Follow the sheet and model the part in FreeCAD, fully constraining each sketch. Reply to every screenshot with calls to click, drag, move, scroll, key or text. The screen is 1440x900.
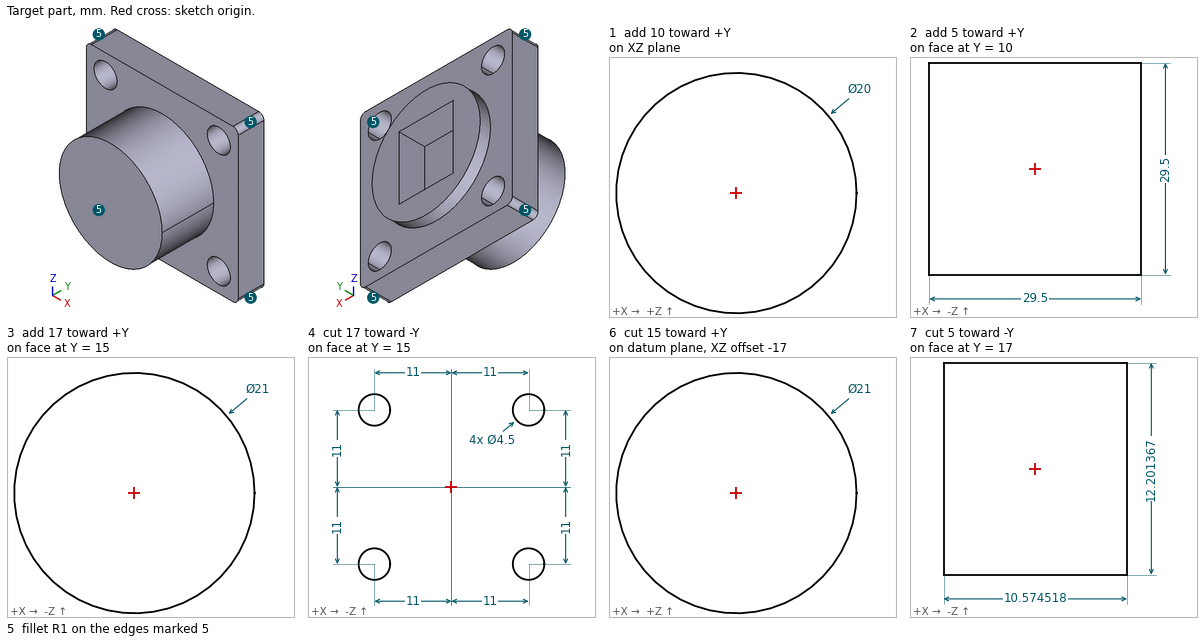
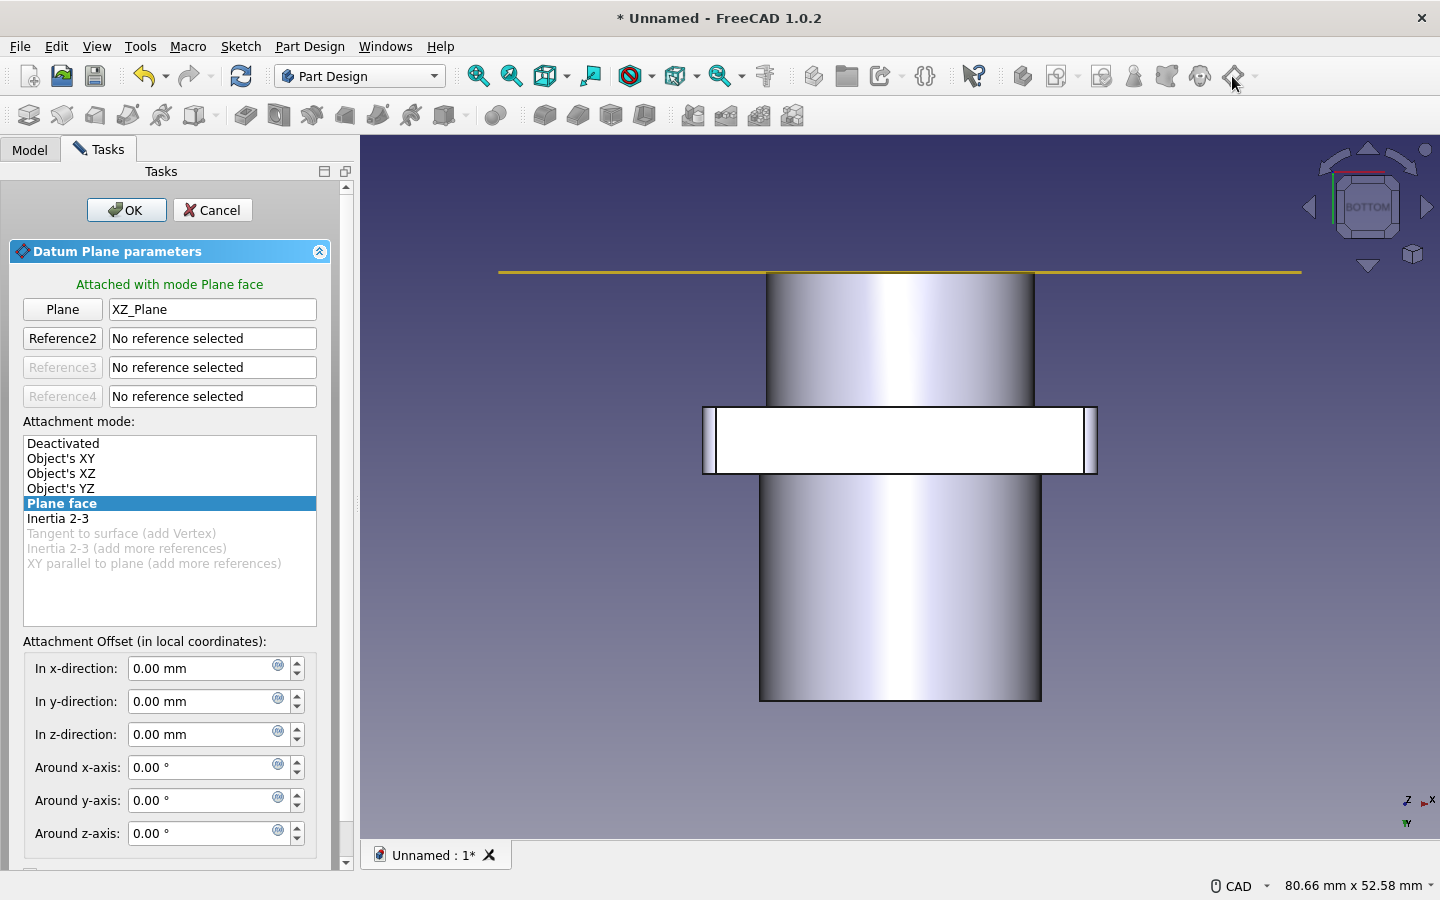
triple_click(210, 734)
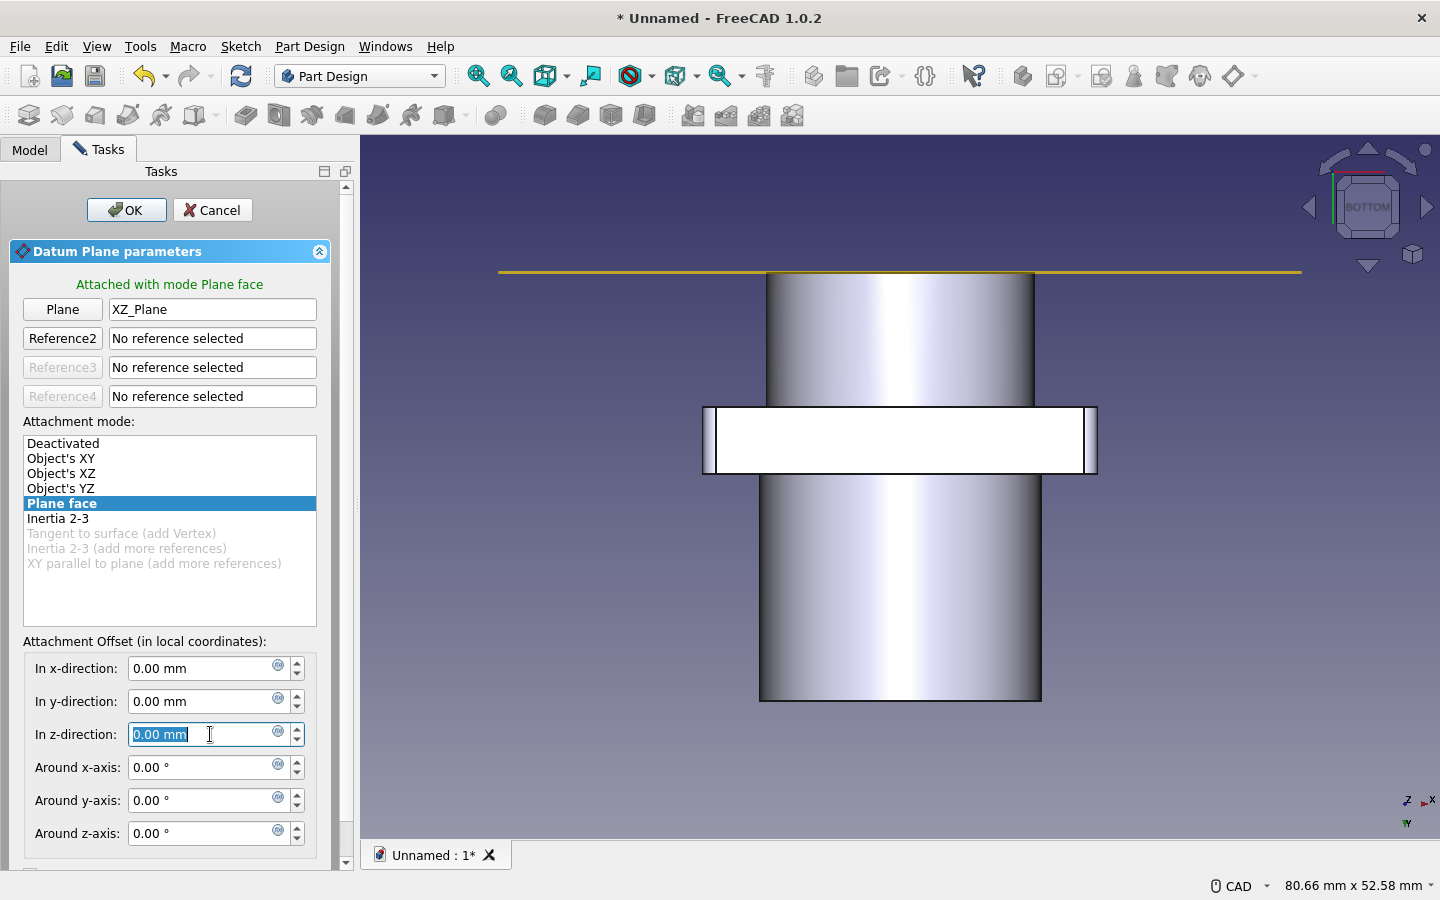
text(-17)
key(Tab)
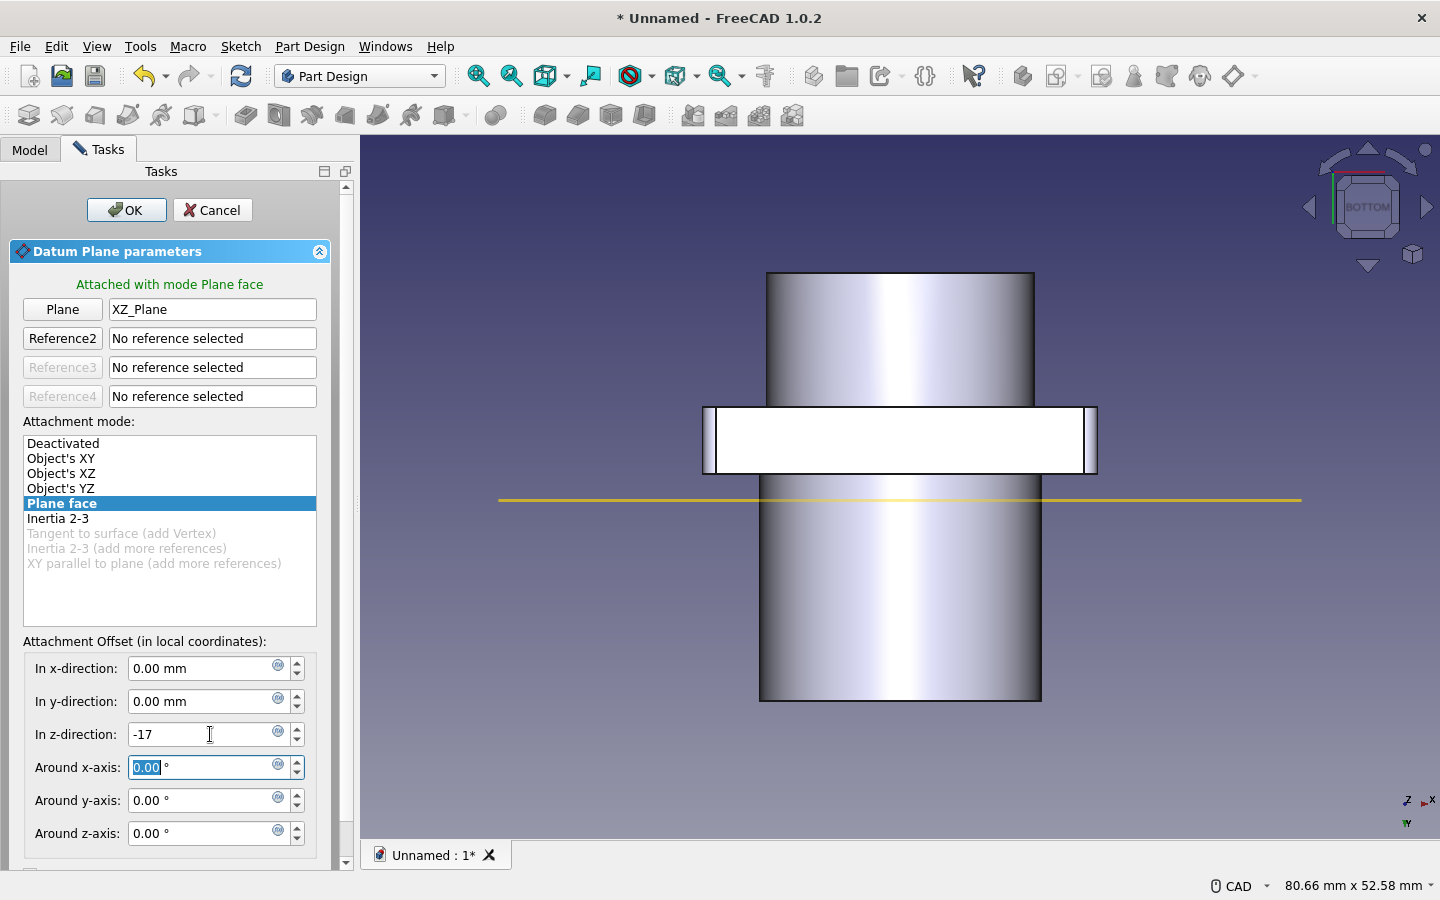
click(127, 210)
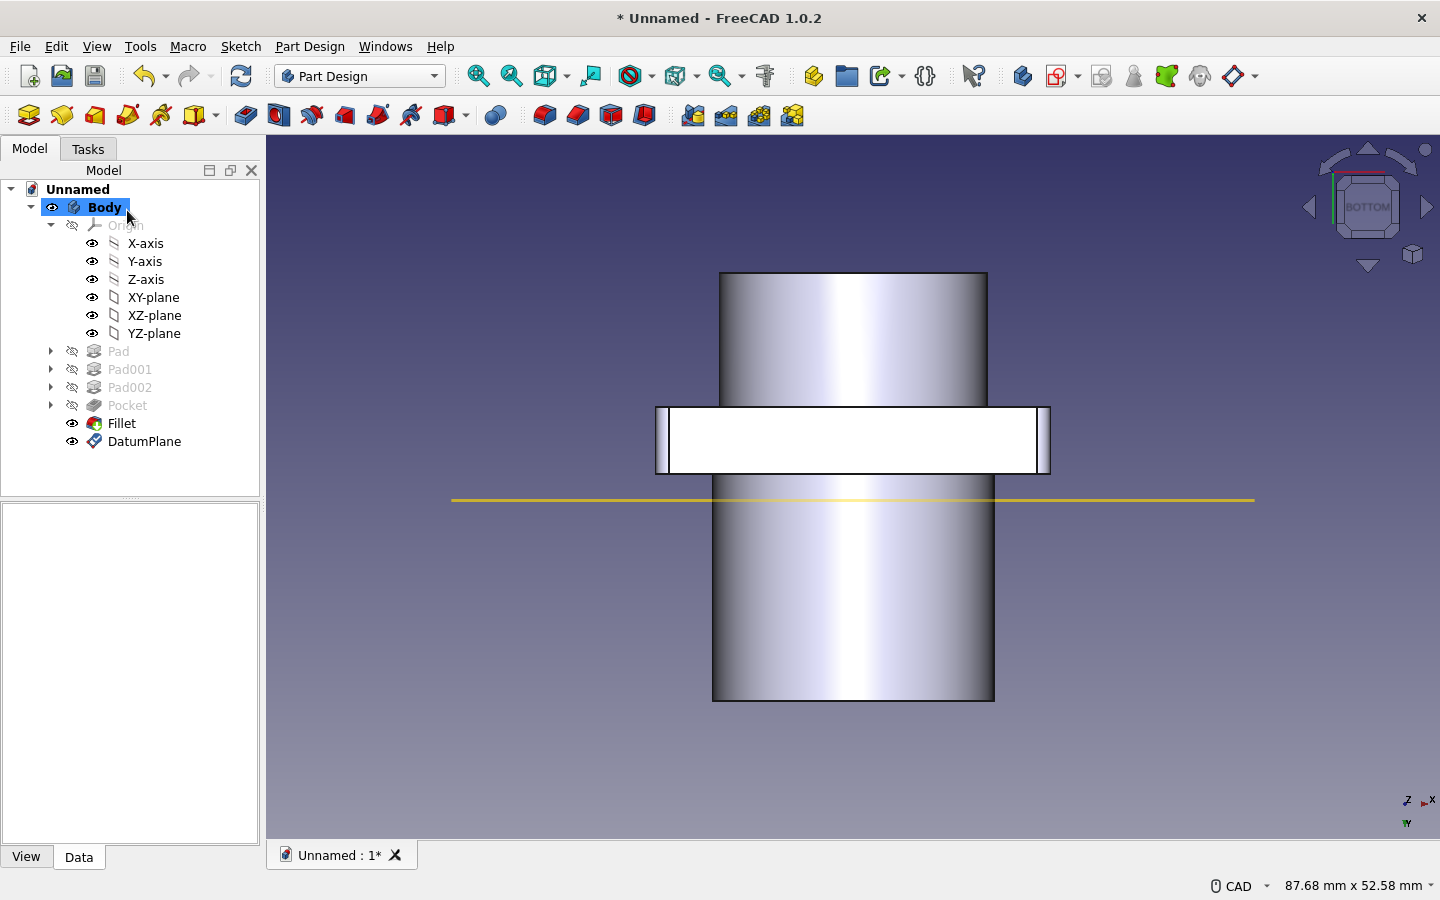
click(117, 441)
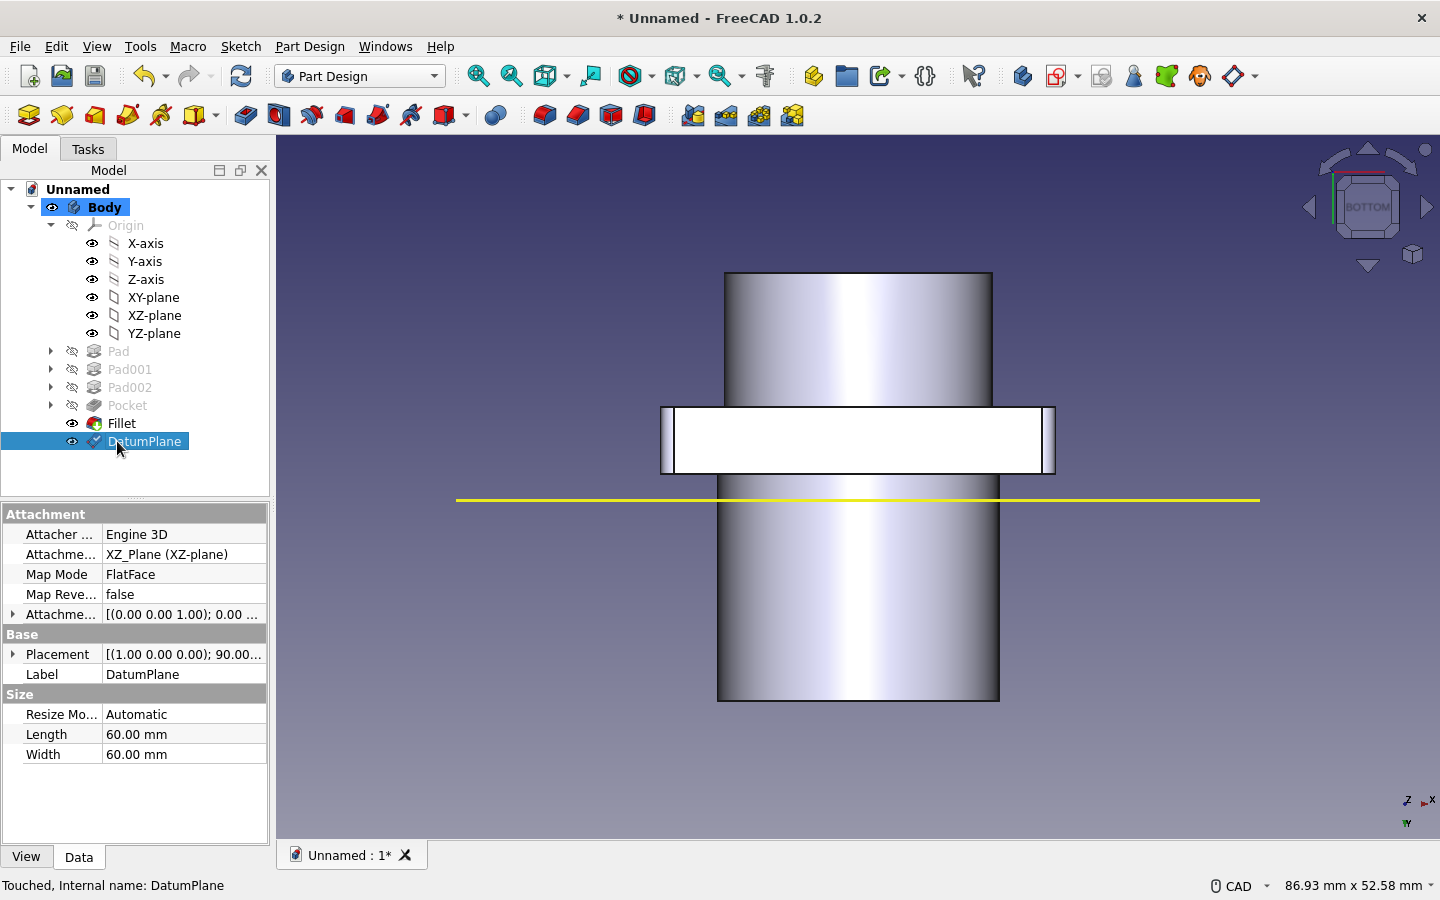
click(1056, 76)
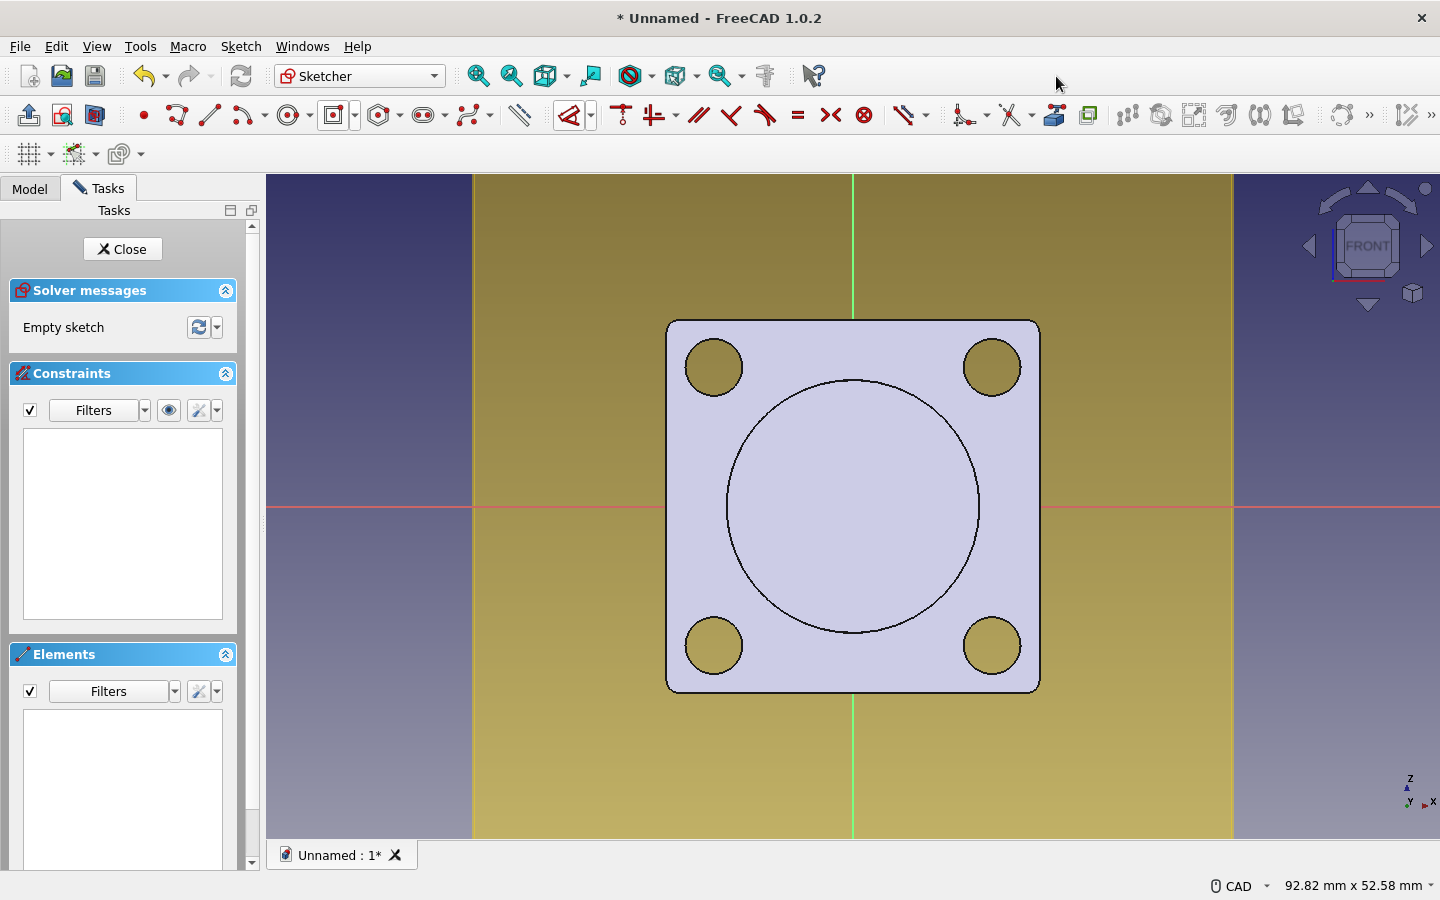
click(95, 116)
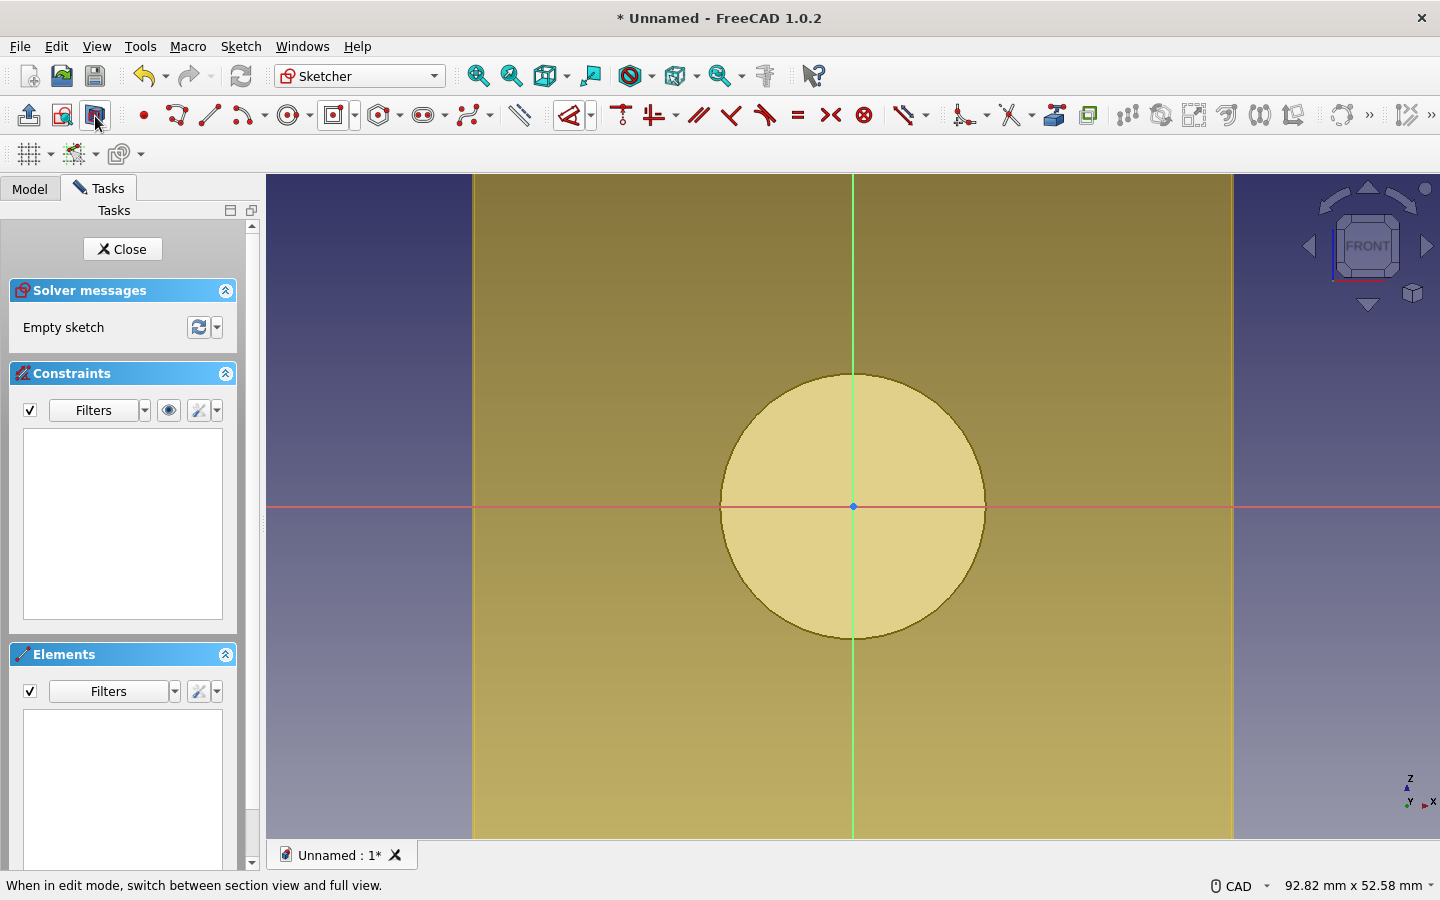
scroll(992, 507, up, 2)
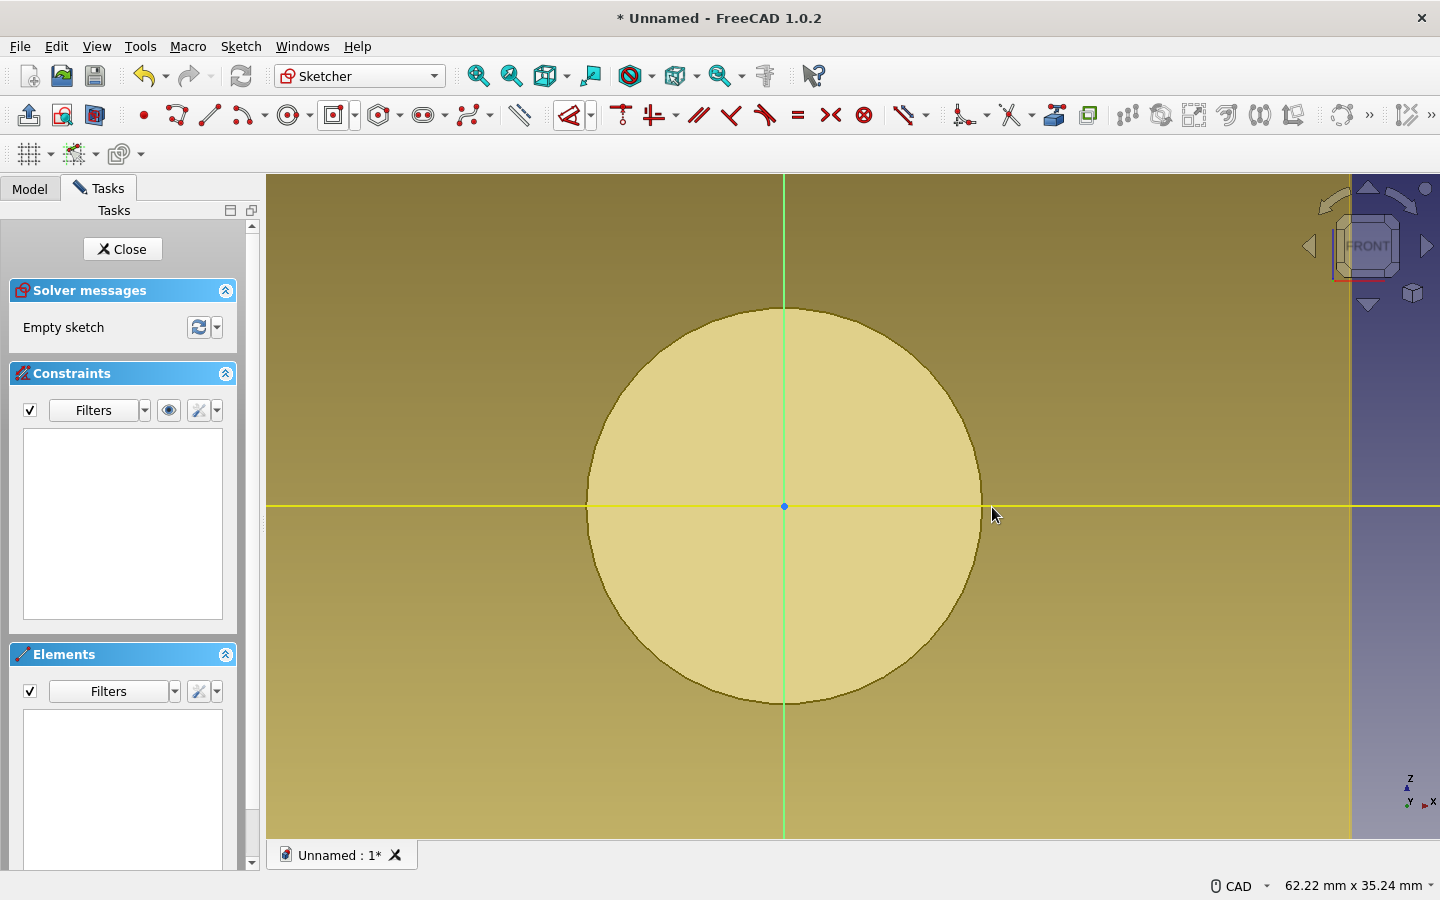
click(288, 116)